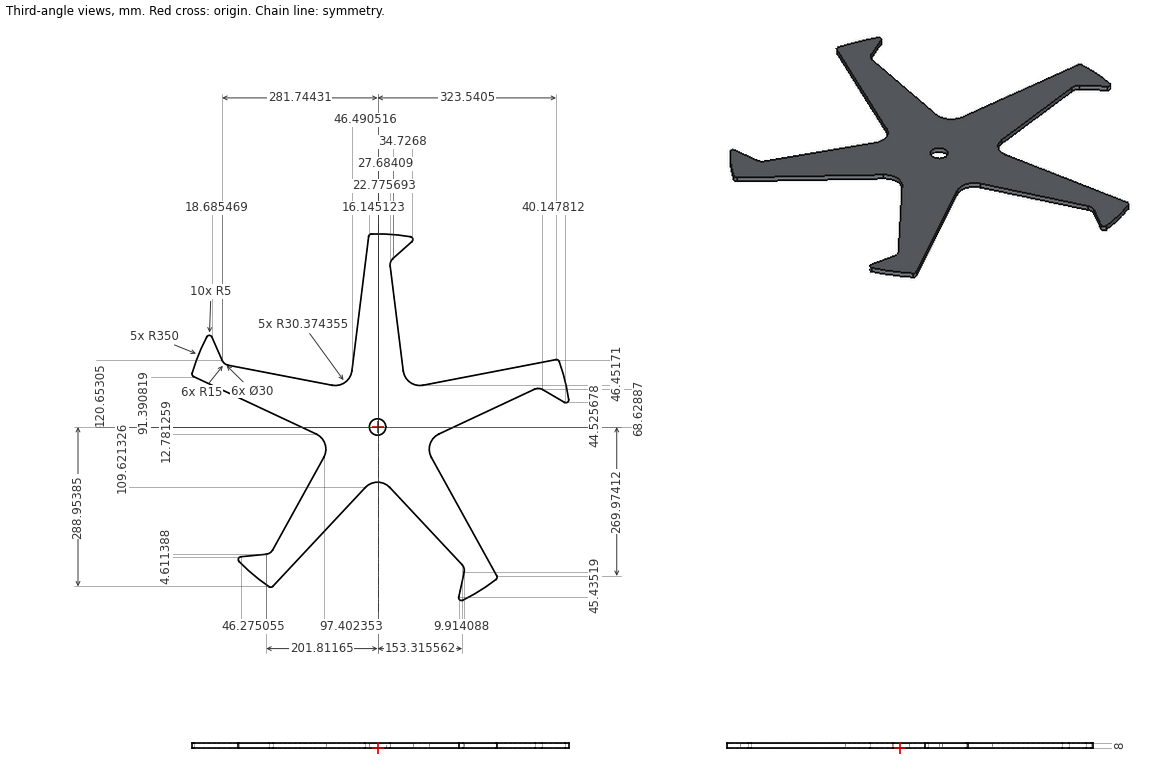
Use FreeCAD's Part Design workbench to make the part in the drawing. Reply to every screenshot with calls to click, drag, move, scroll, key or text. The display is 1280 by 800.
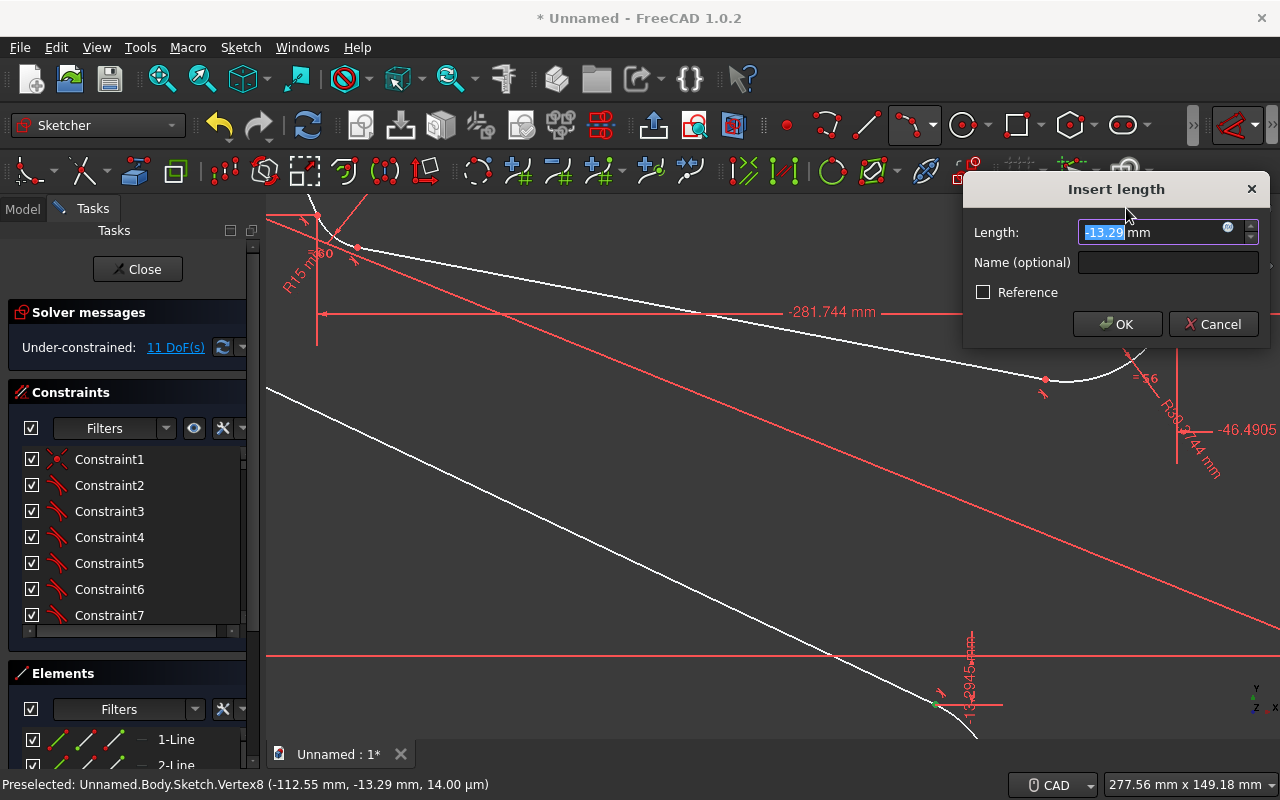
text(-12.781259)
key(Return)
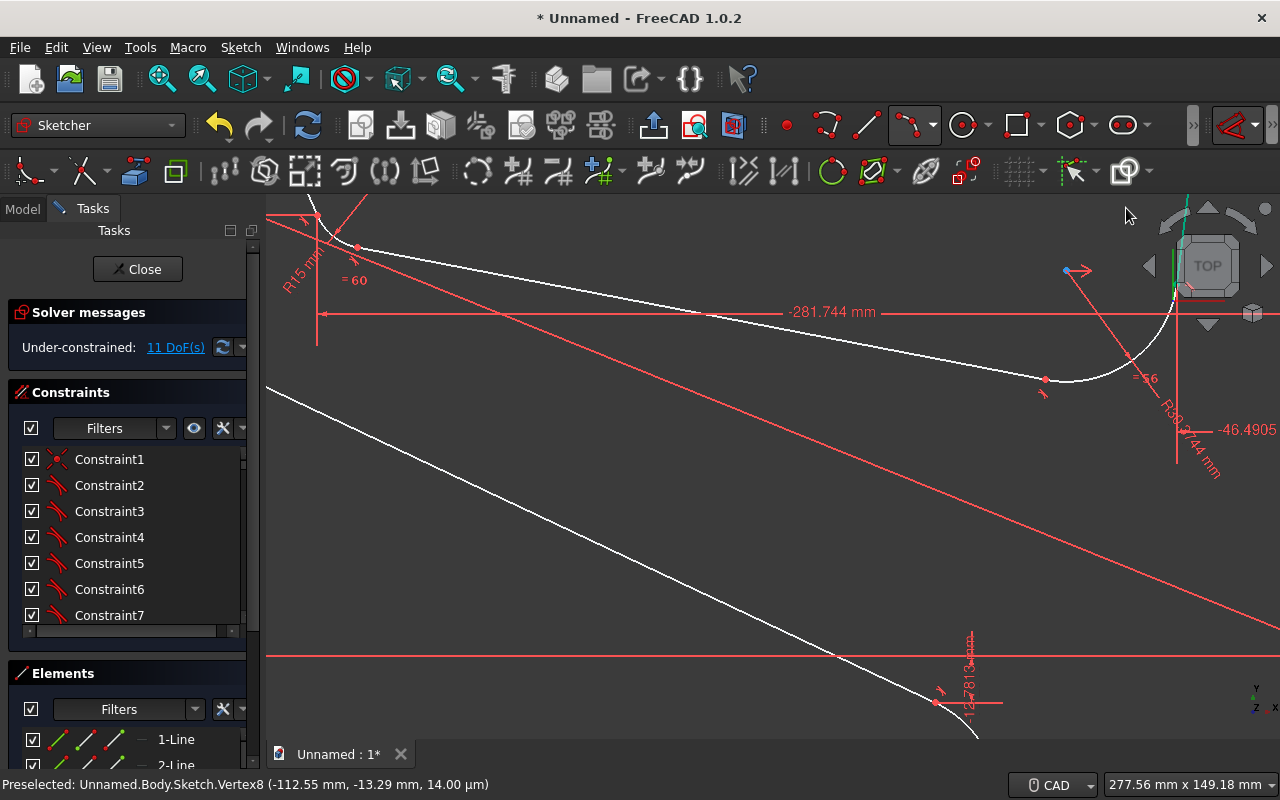
scroll(601, 447, down, 10)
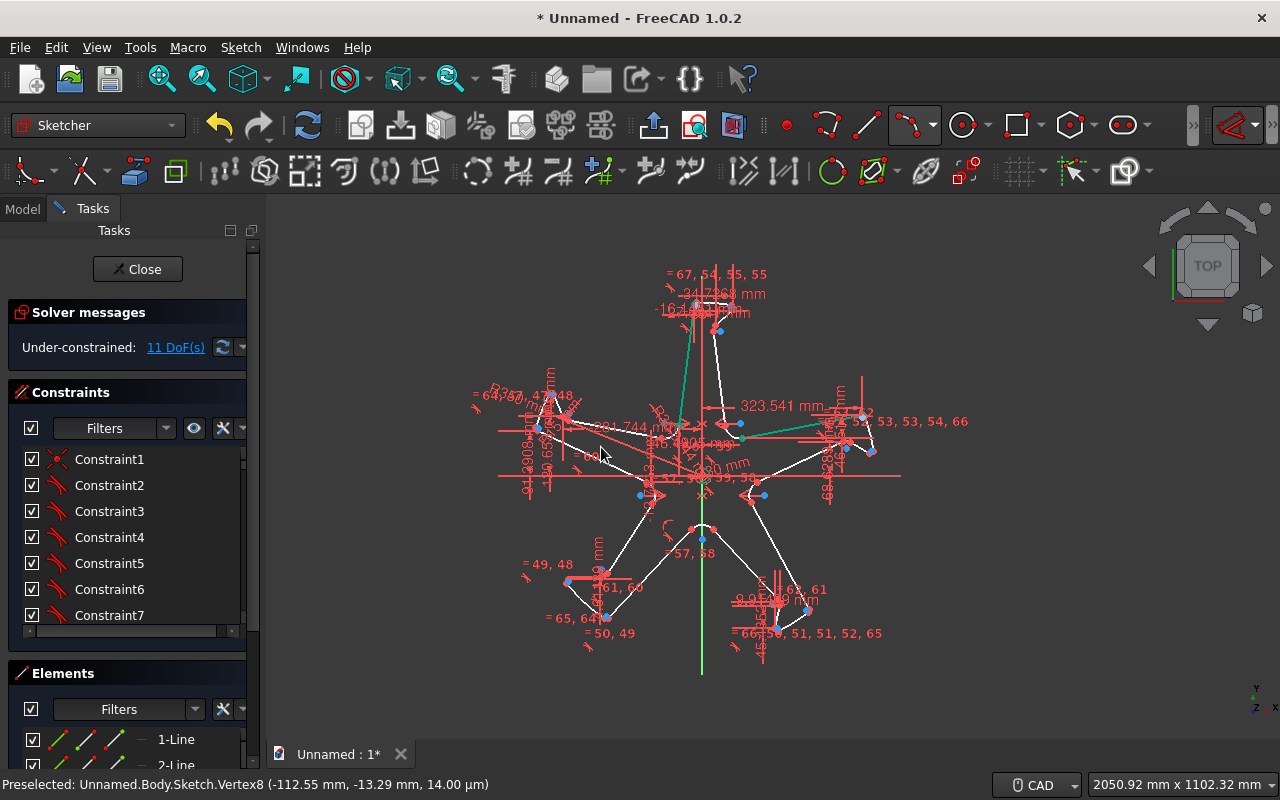
click(653, 504)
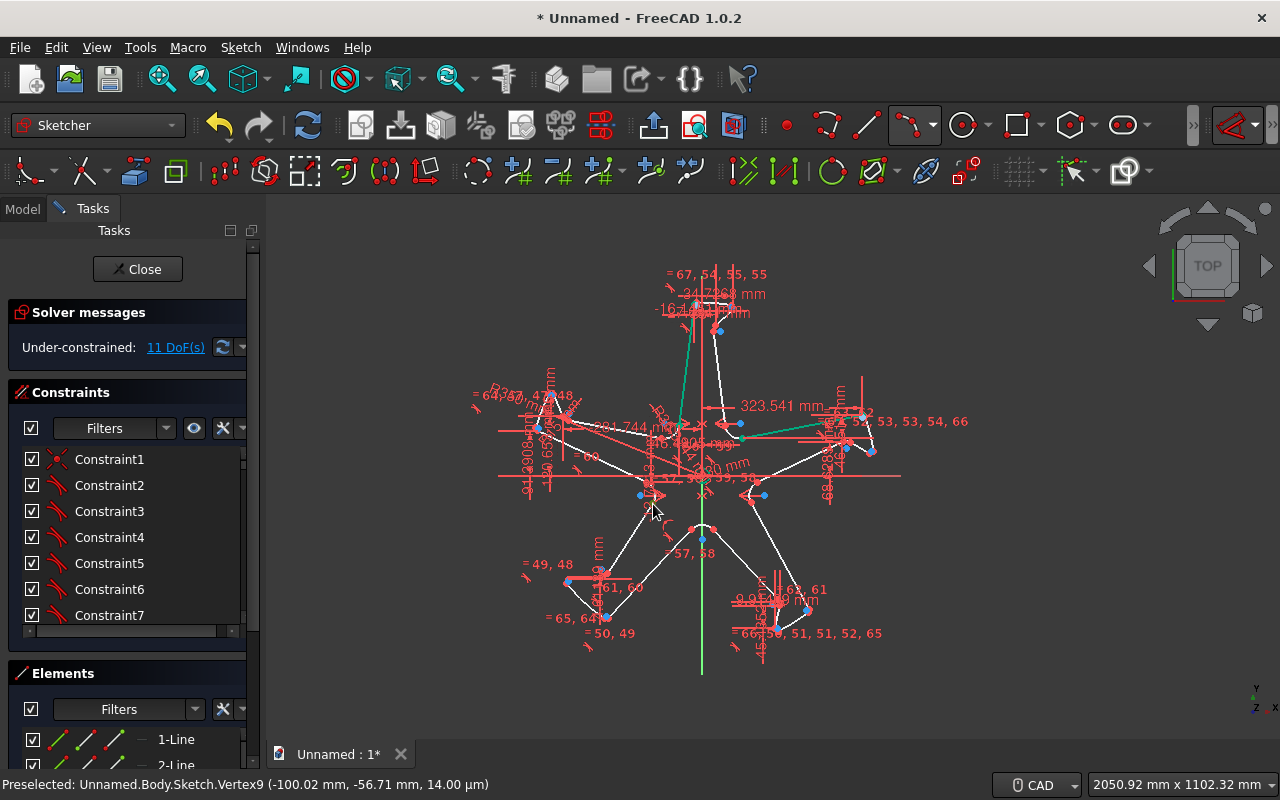
key(l)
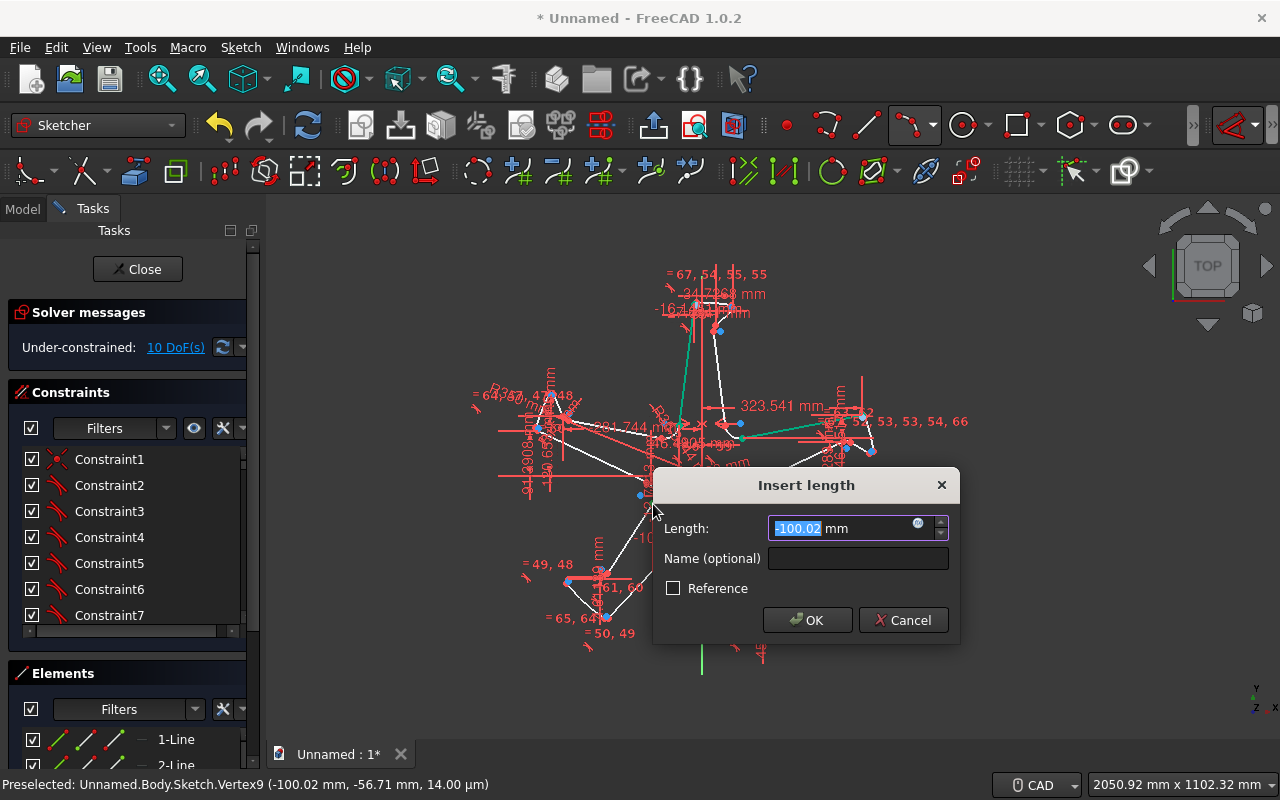
text(-97.402353)
key(Return)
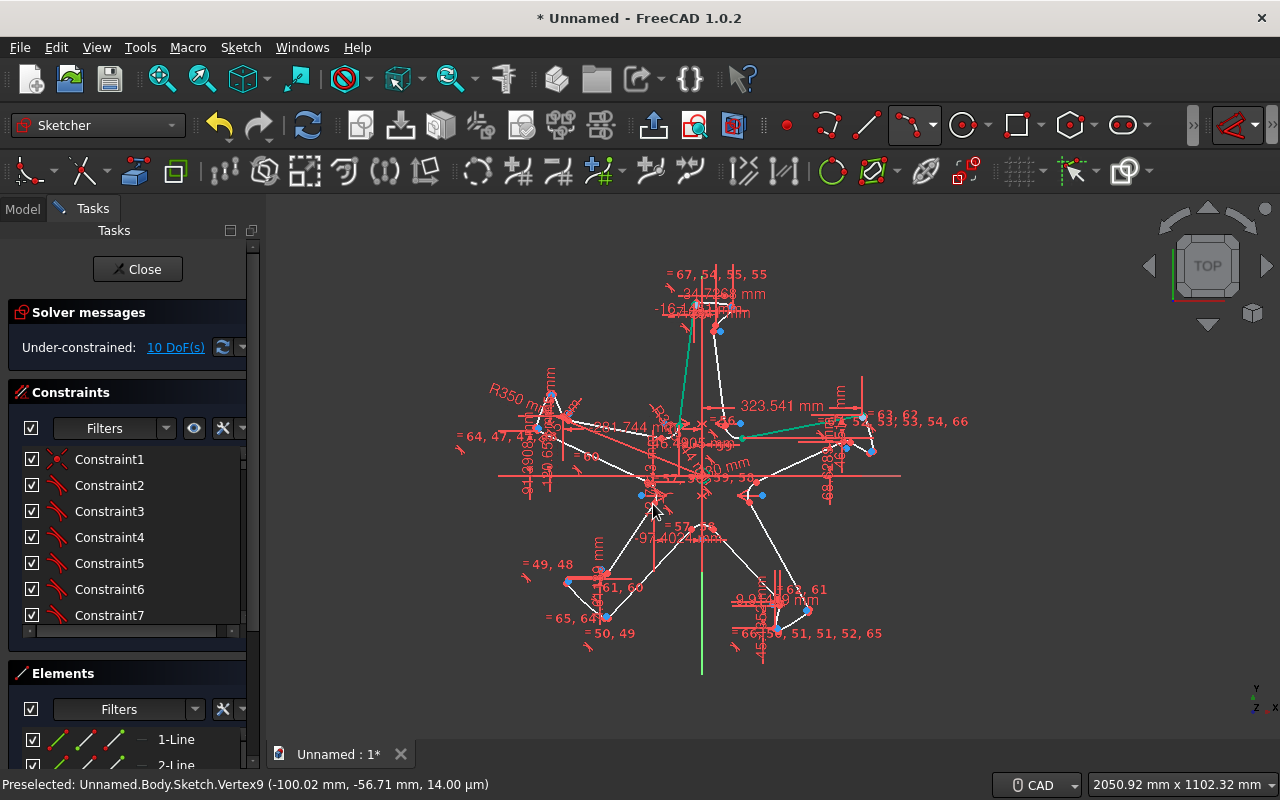
scroll(602, 577, up, 4)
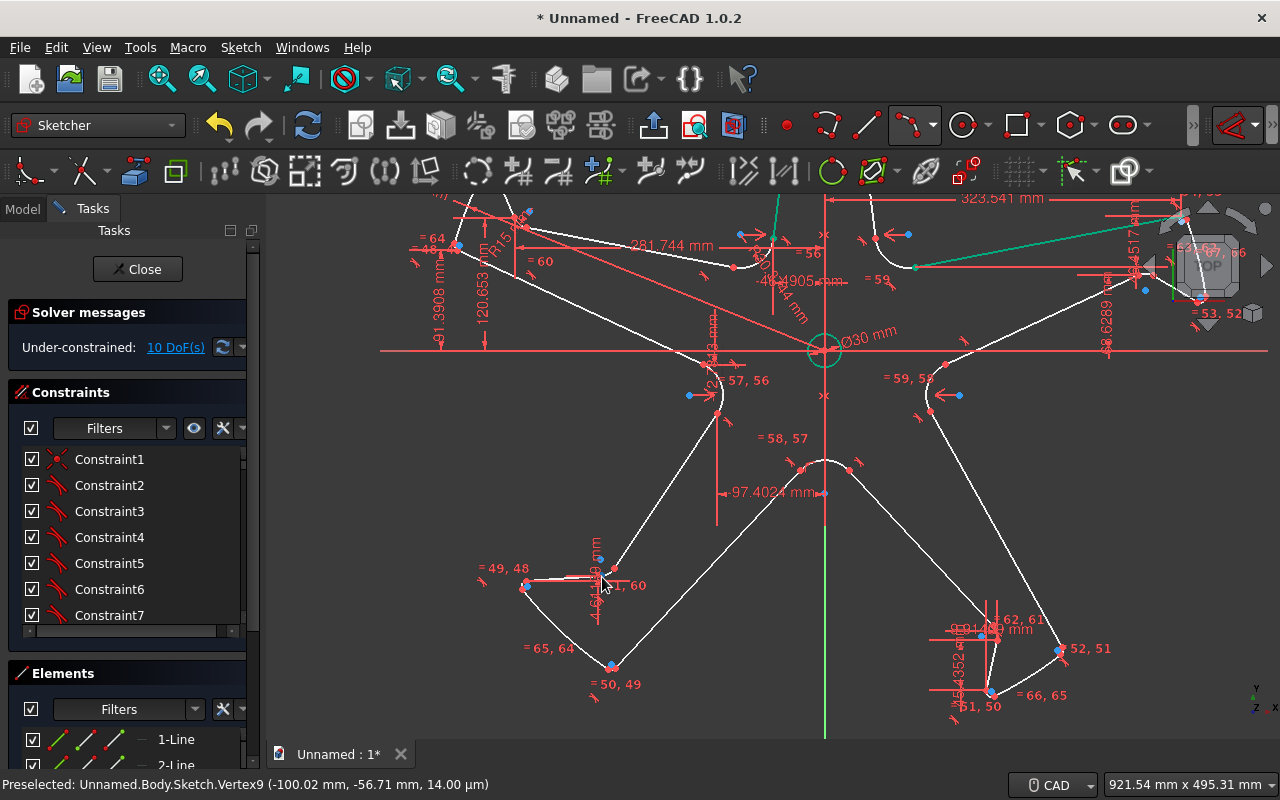
click(602, 576)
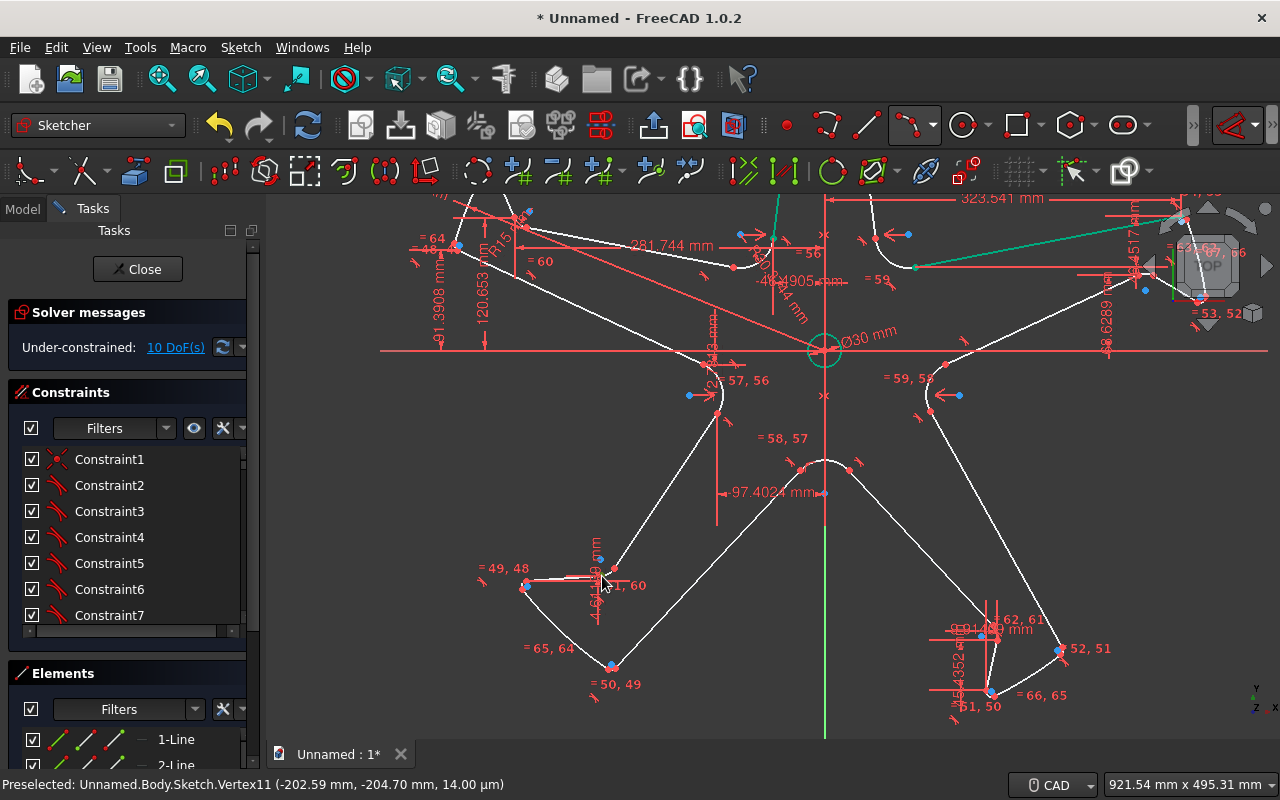
click(1258, 126)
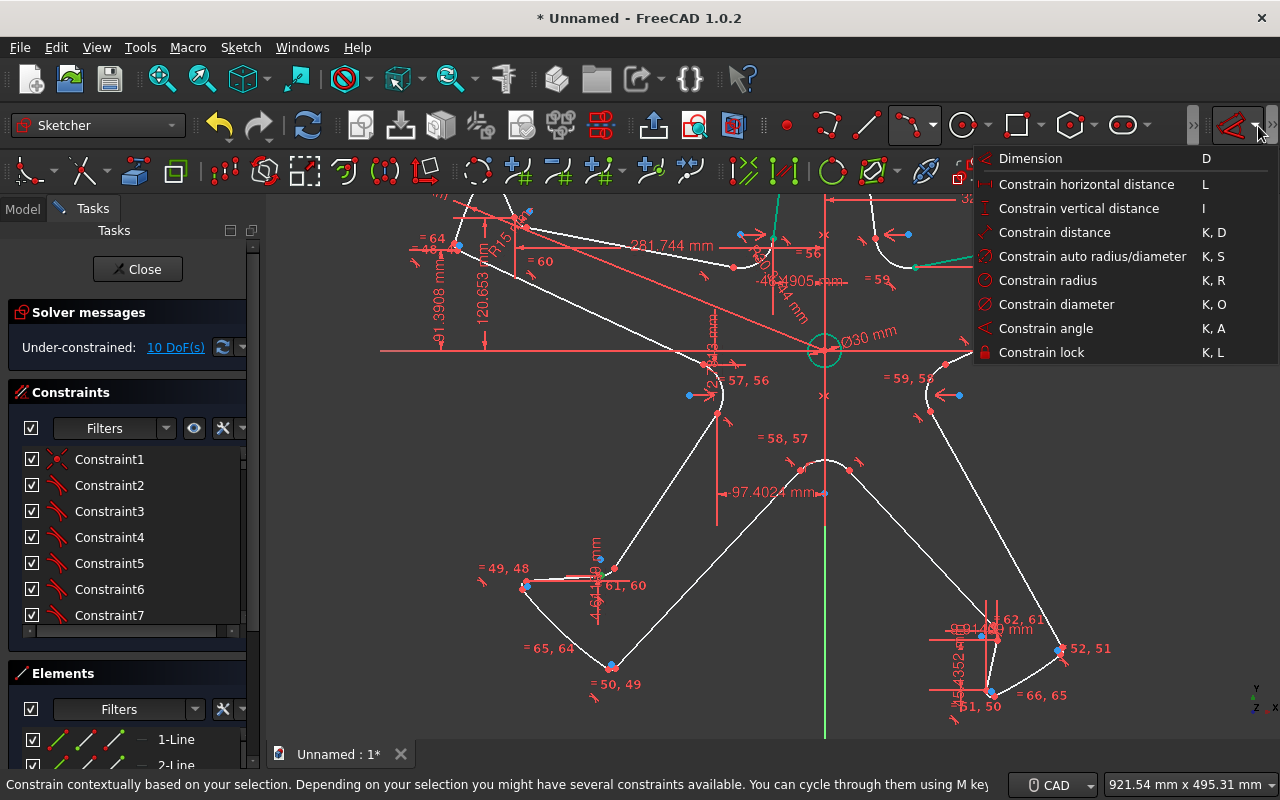
click(1126, 184)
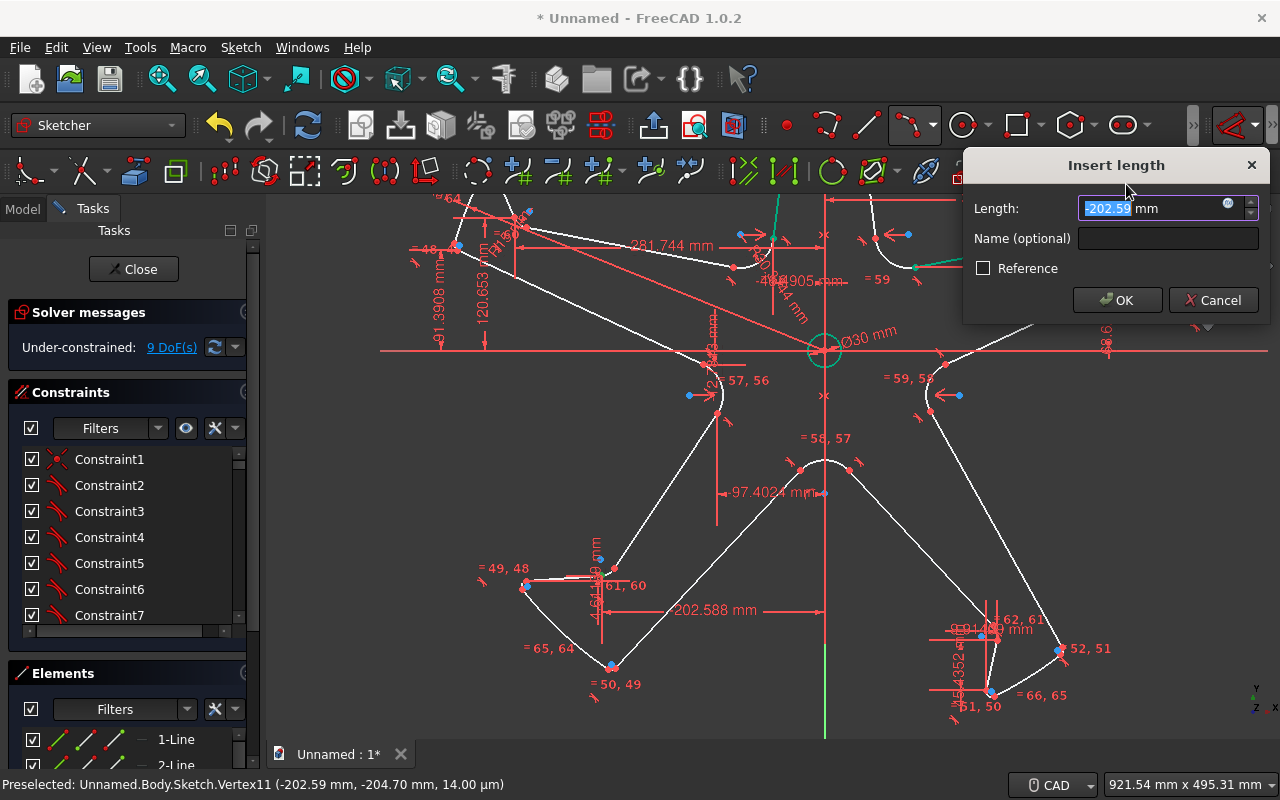
text(-201.81165)
key(Return)